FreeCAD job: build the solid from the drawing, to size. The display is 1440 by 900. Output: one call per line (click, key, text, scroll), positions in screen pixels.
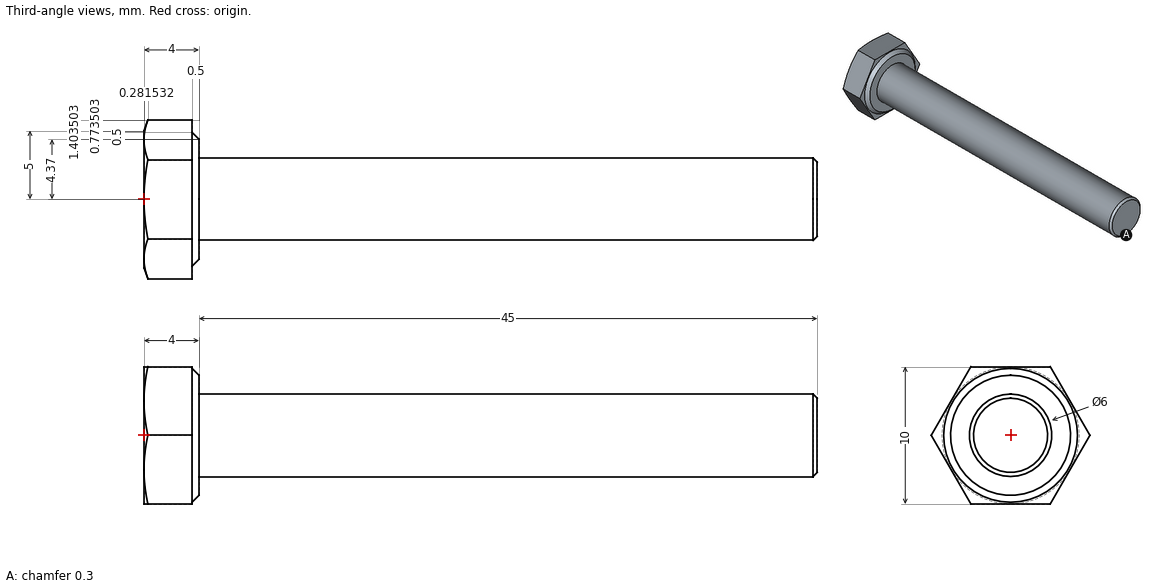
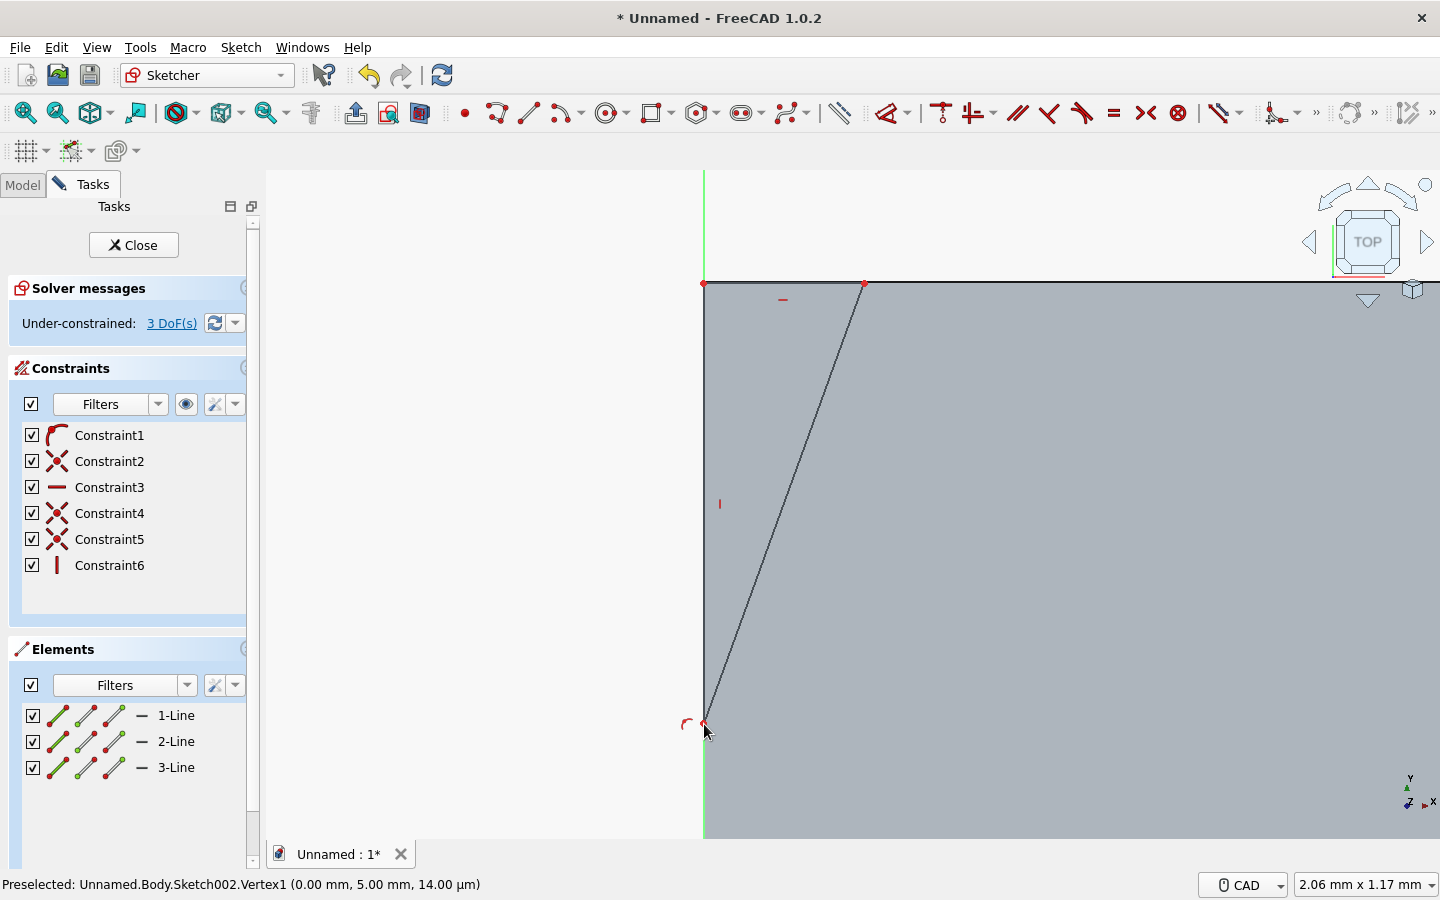
click(886, 114)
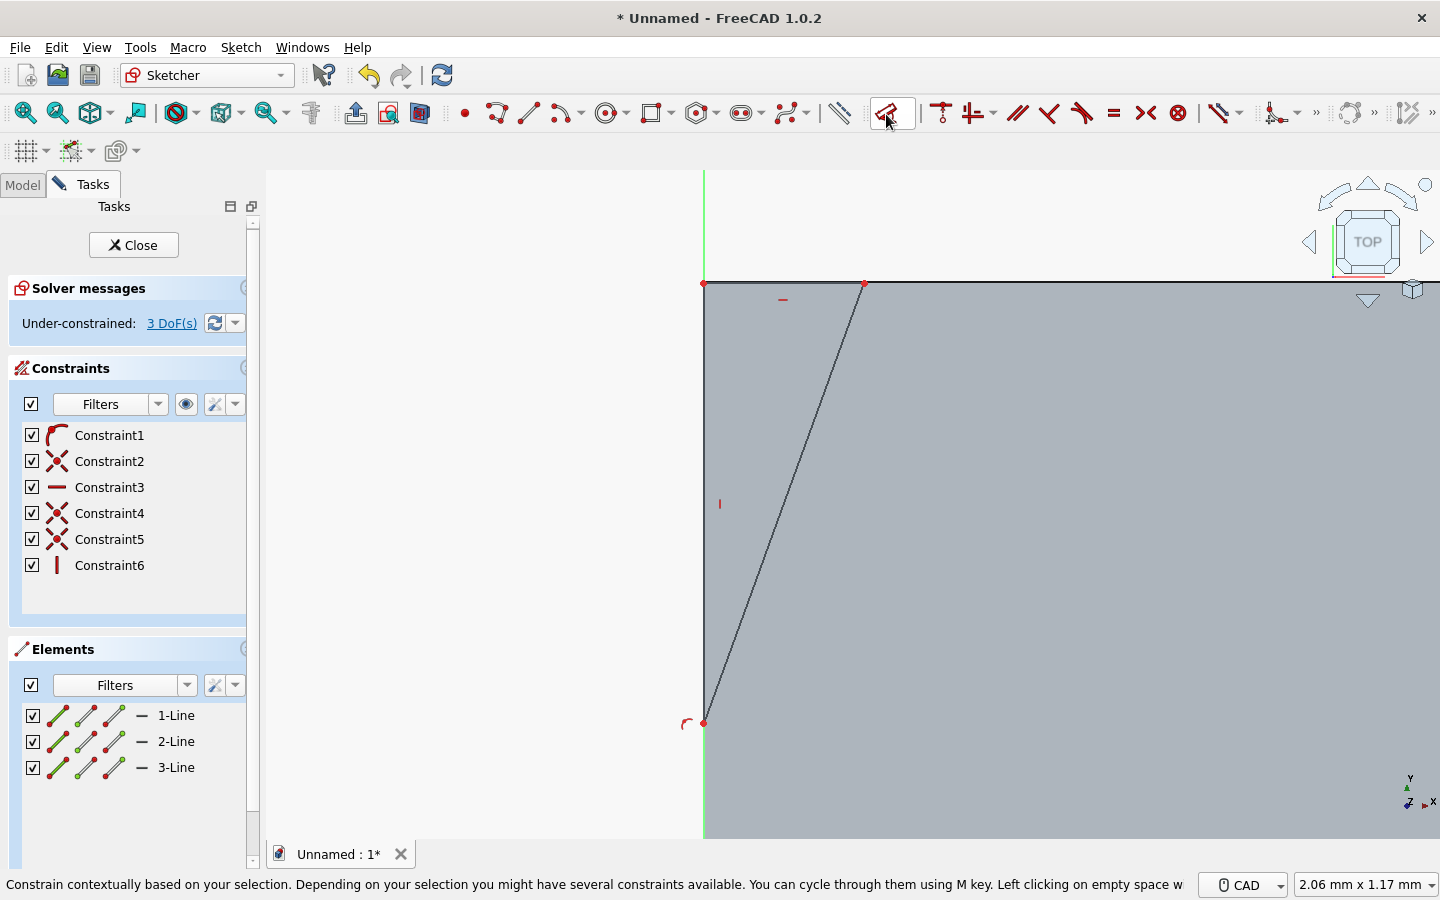
click(704, 724)
click(670, 767)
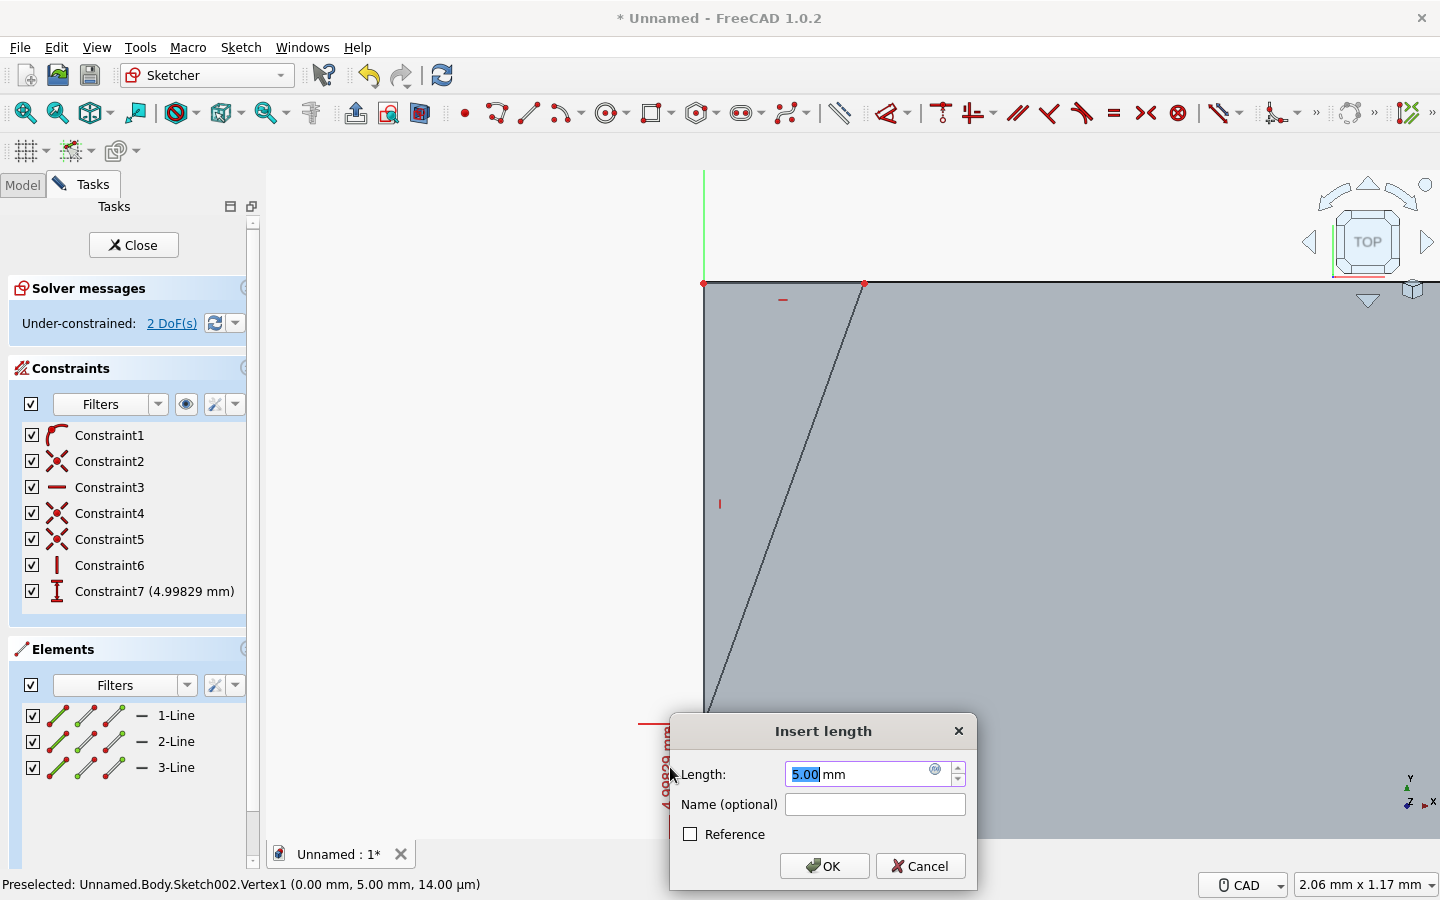
text(5)
key(Return)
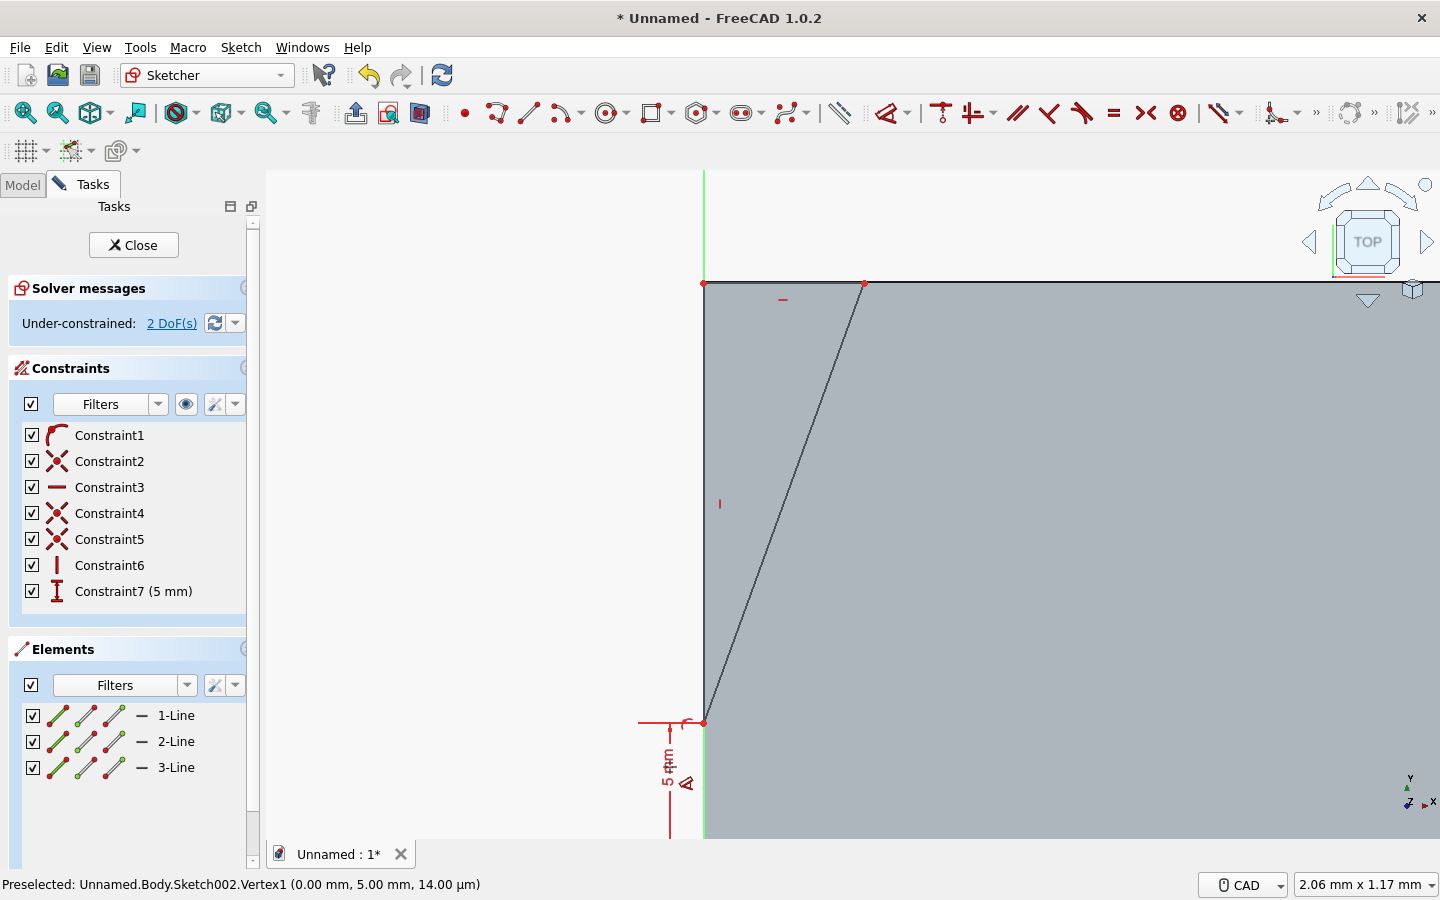
click(816, 283)
click(784, 249)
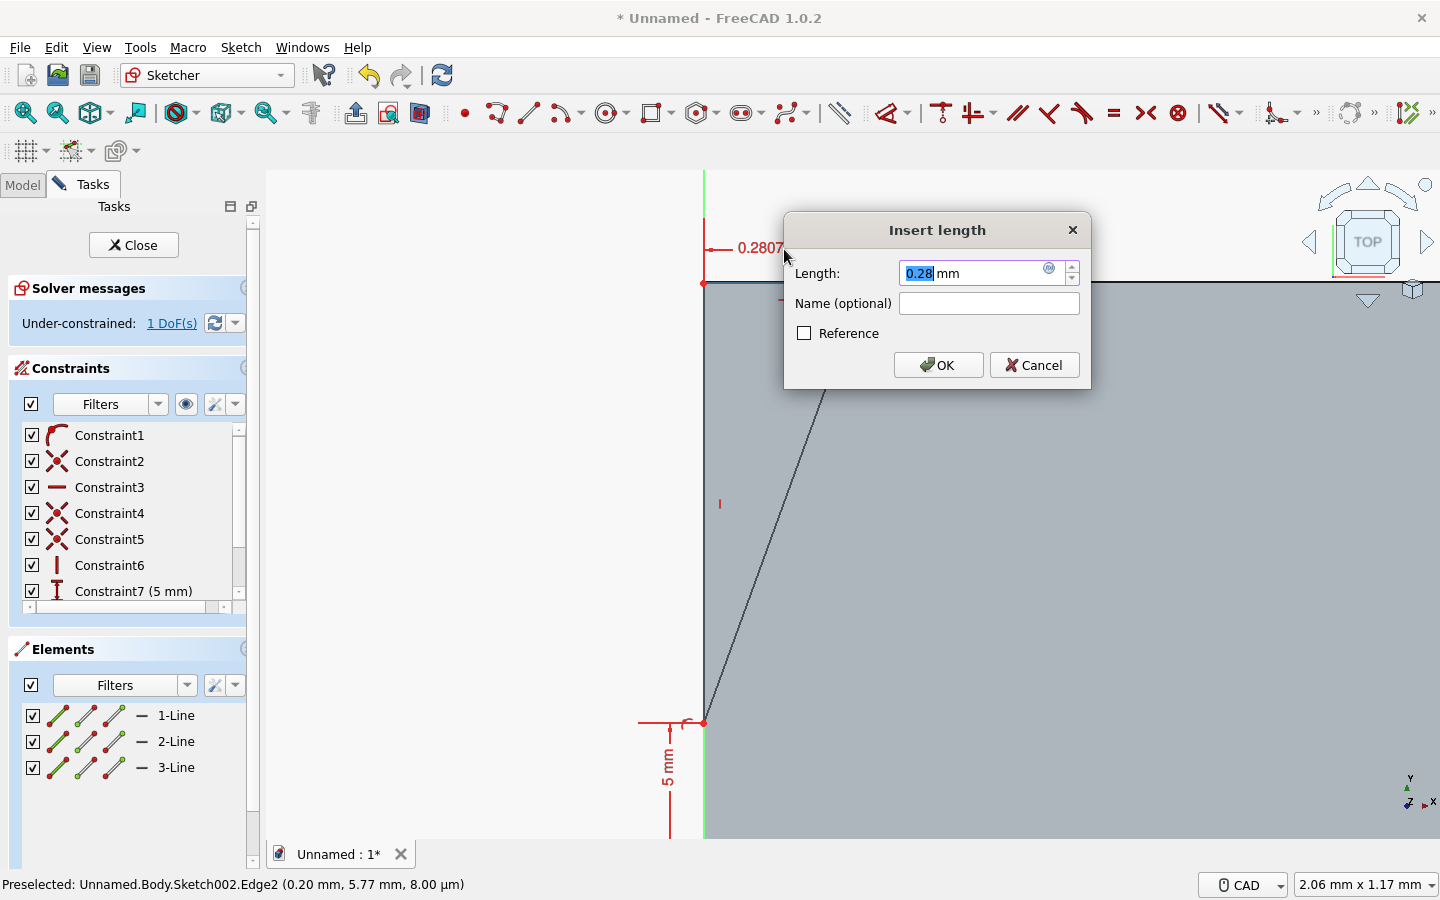
text(0.281532)
key(Return)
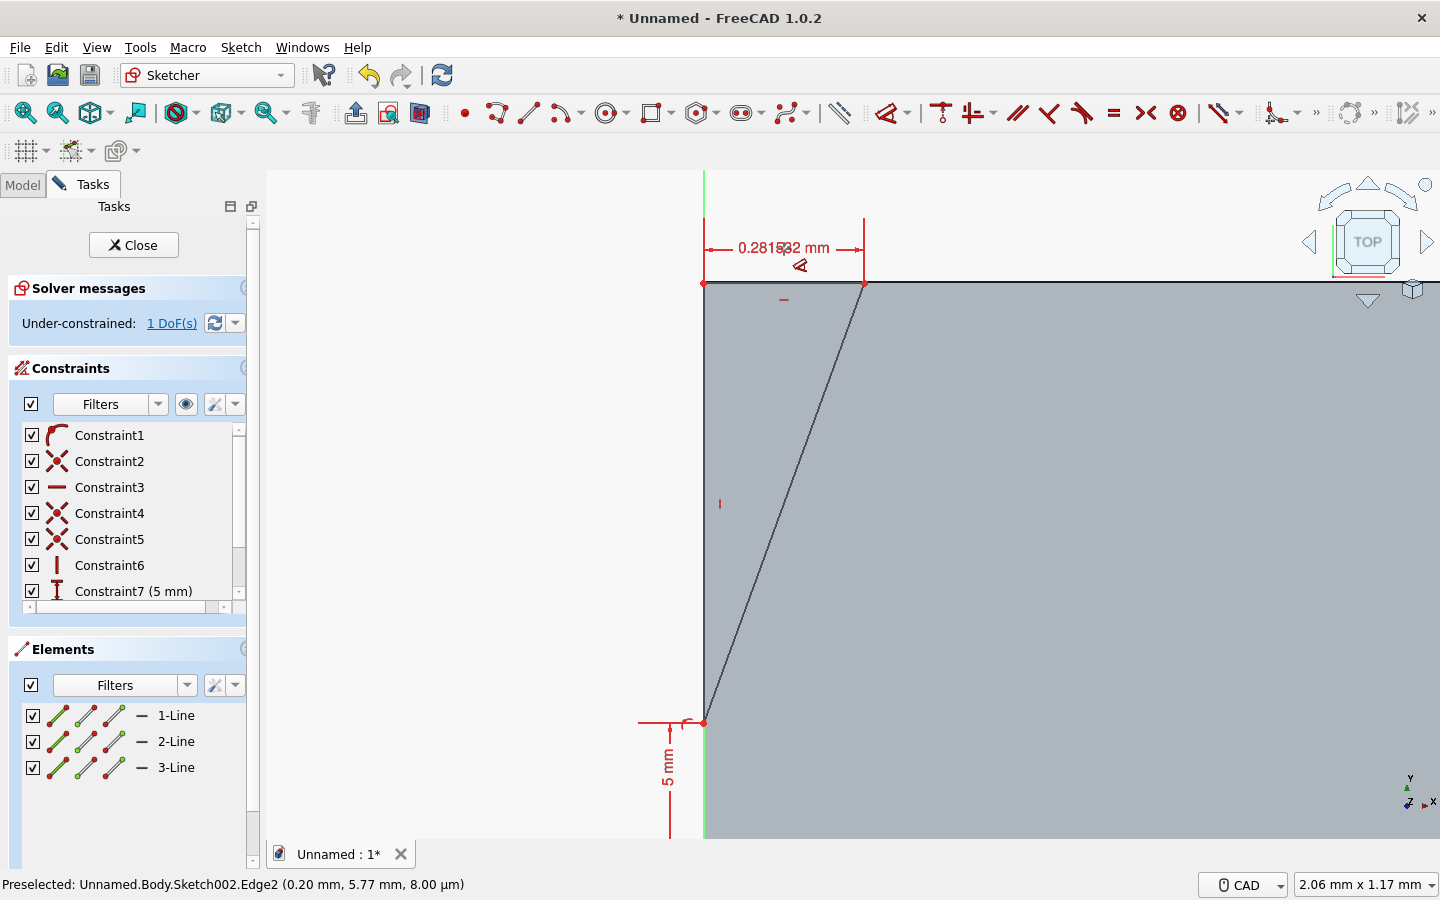
click(704, 415)
click(670, 503)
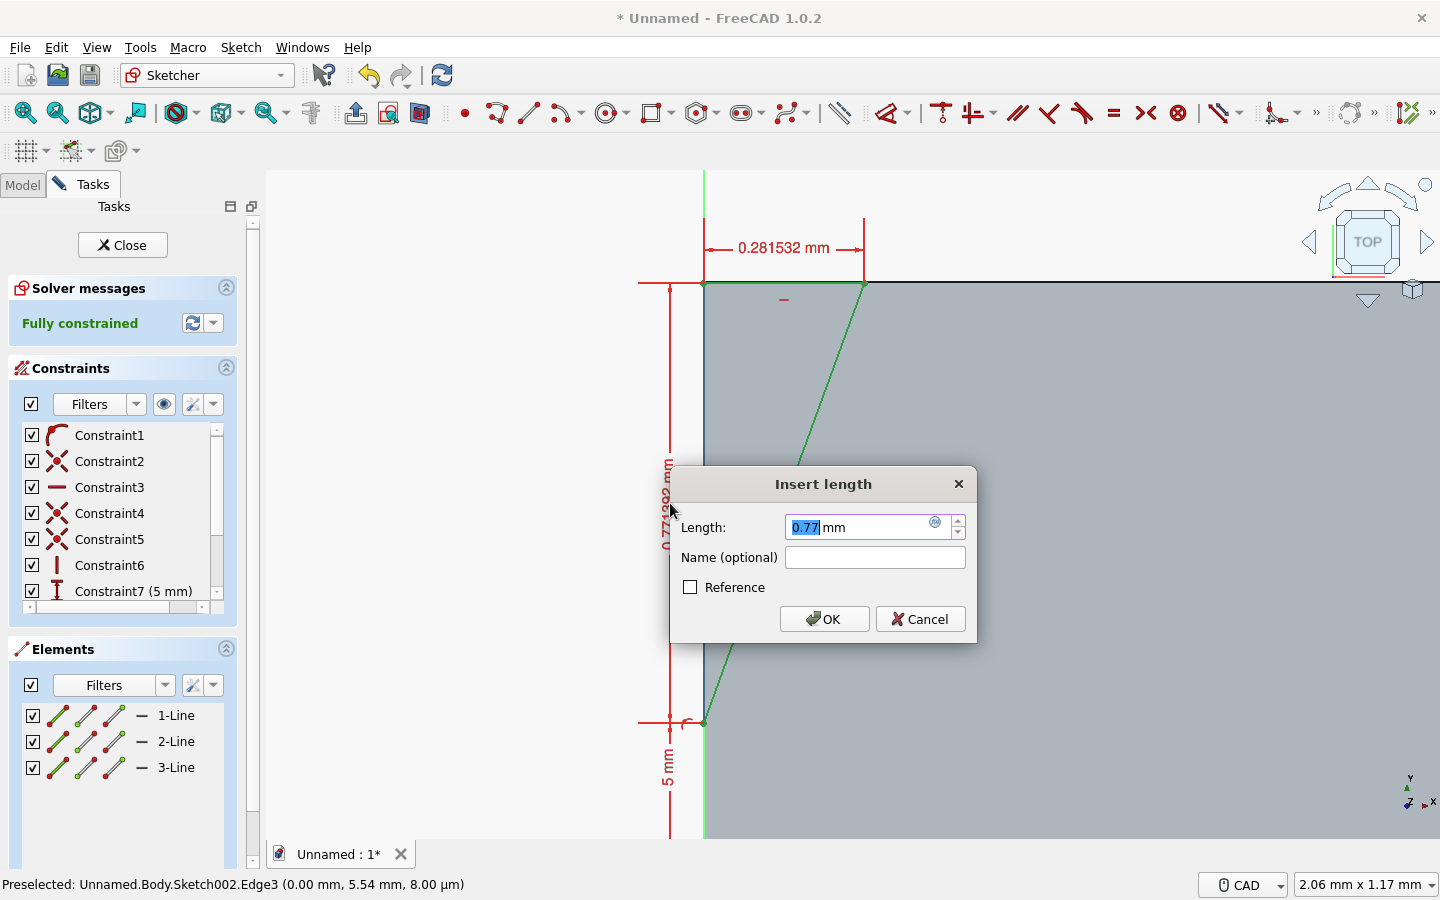
text(0.773503)
key(Return)
key(Escape)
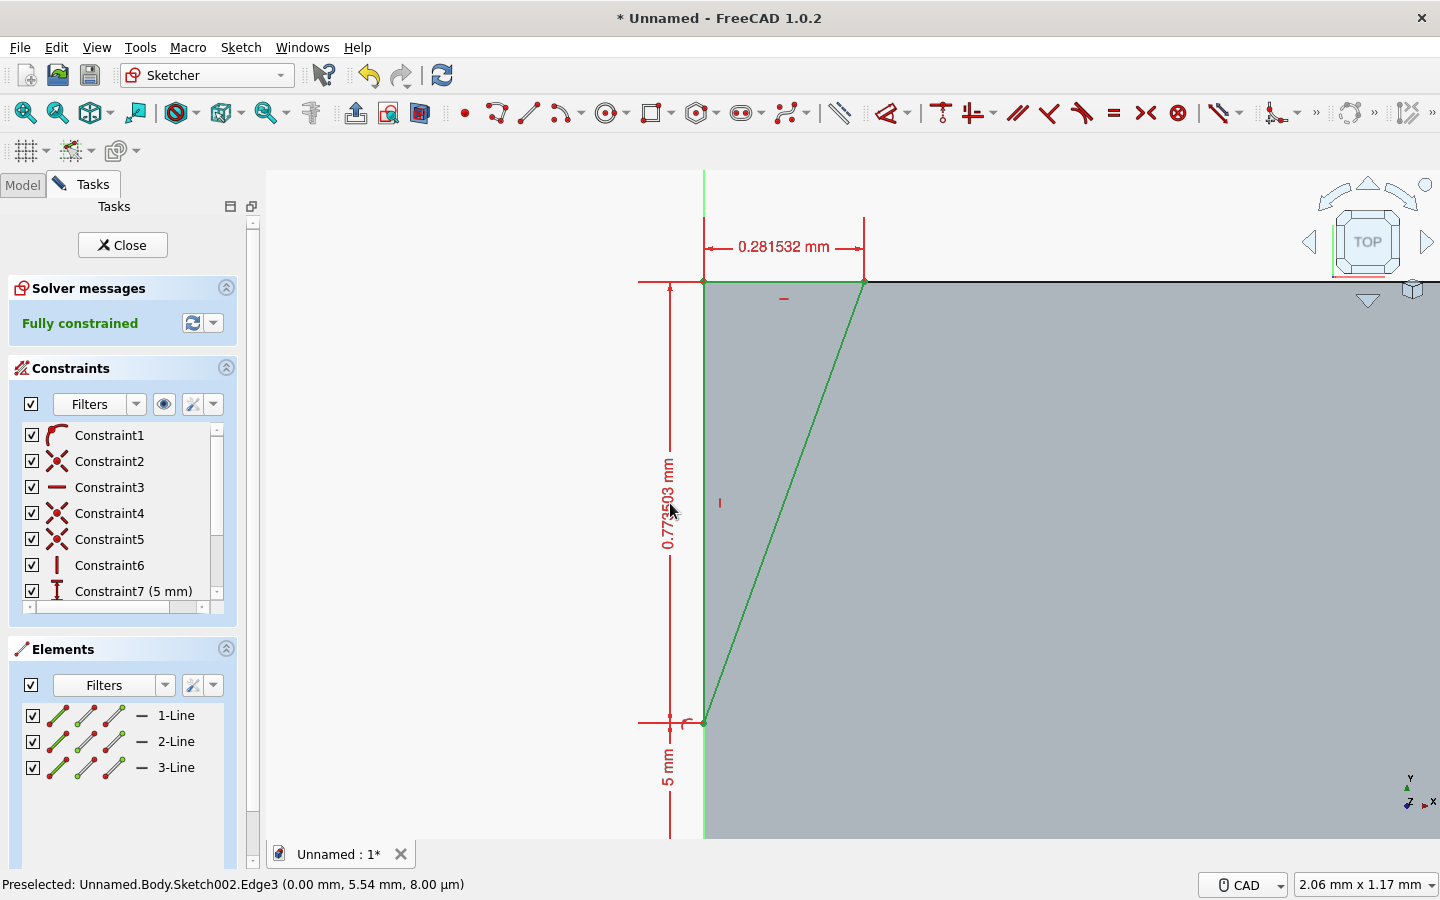
click(123, 245)